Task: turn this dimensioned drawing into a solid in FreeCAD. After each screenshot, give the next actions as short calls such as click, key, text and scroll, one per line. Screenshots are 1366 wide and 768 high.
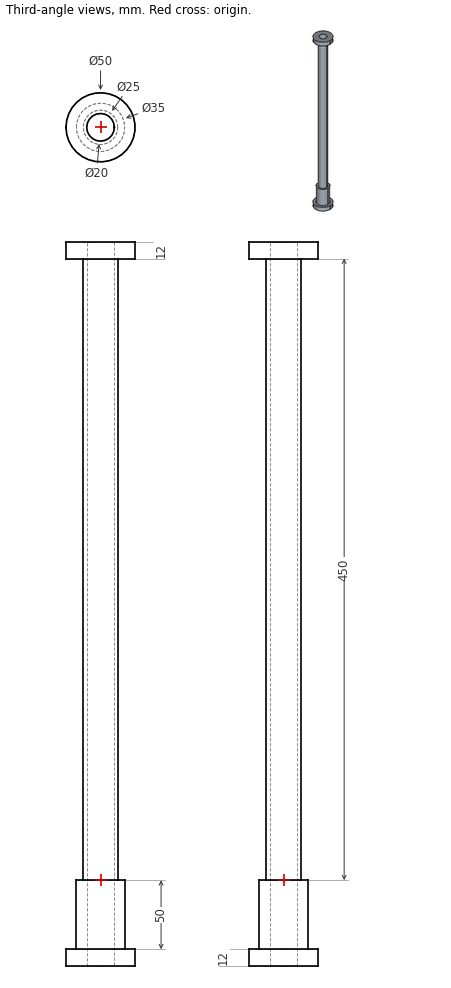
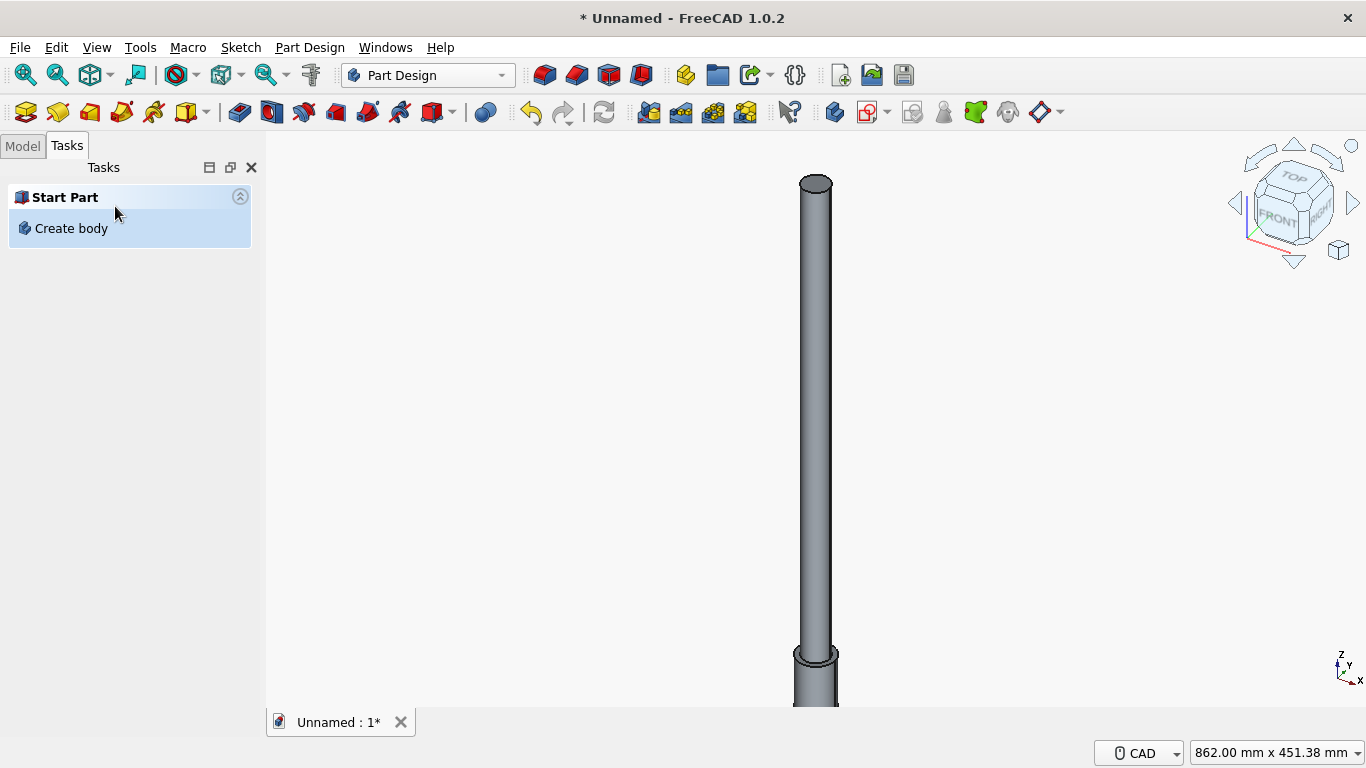
click(26, 76)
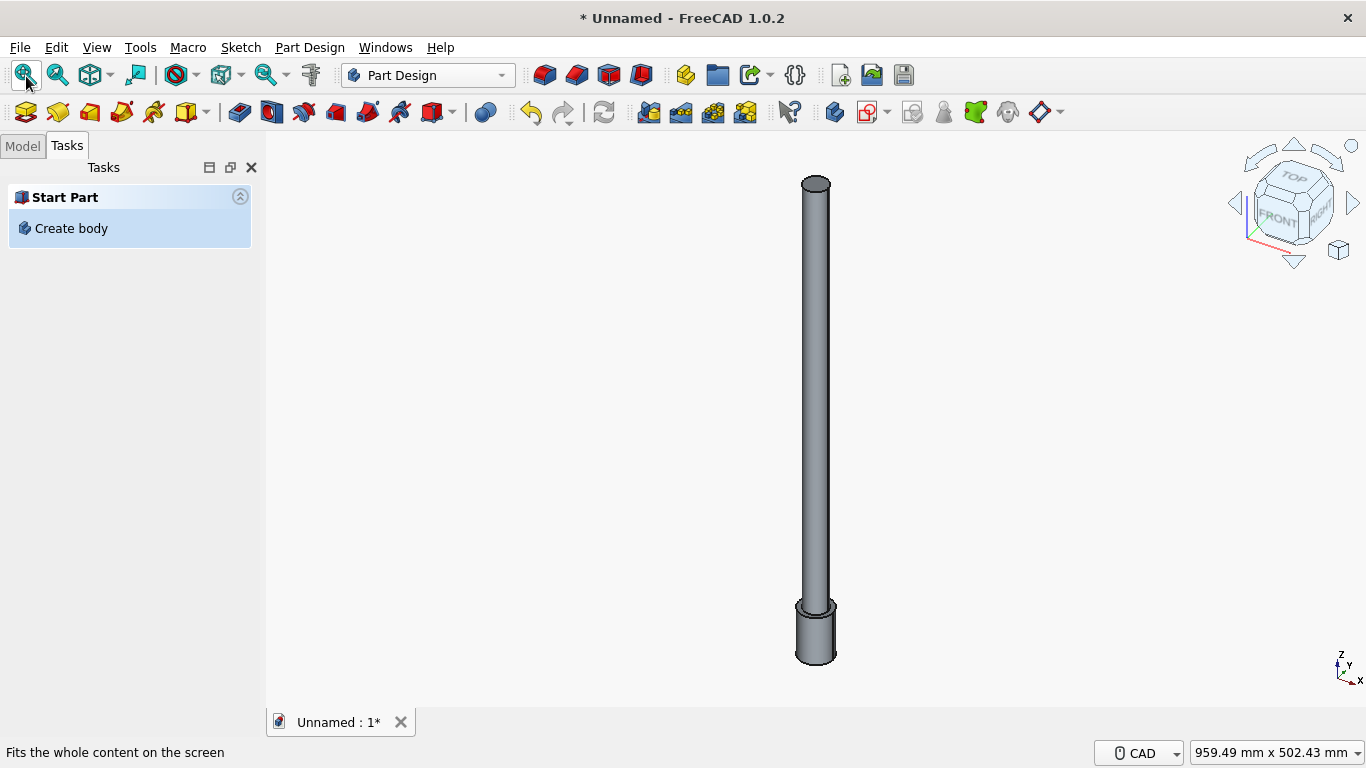
key(5)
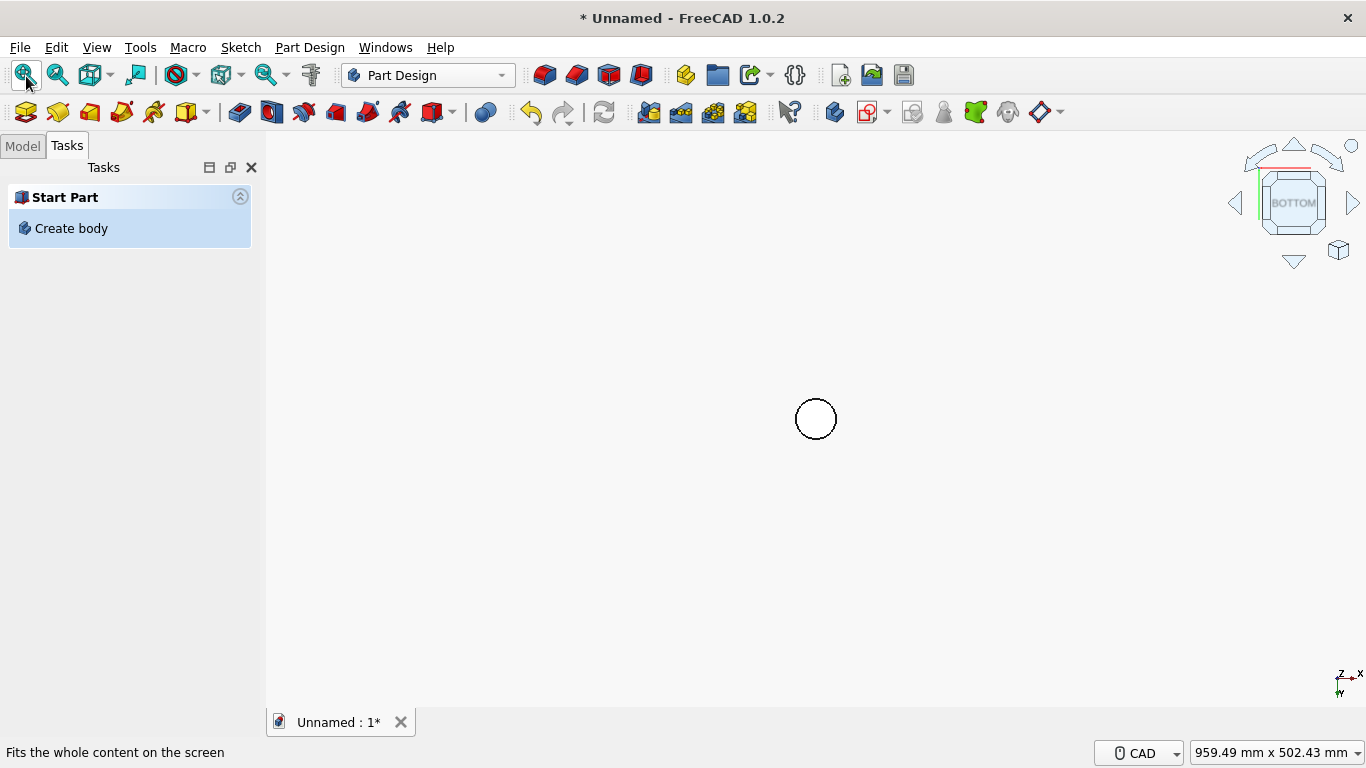
key(v)
key(f)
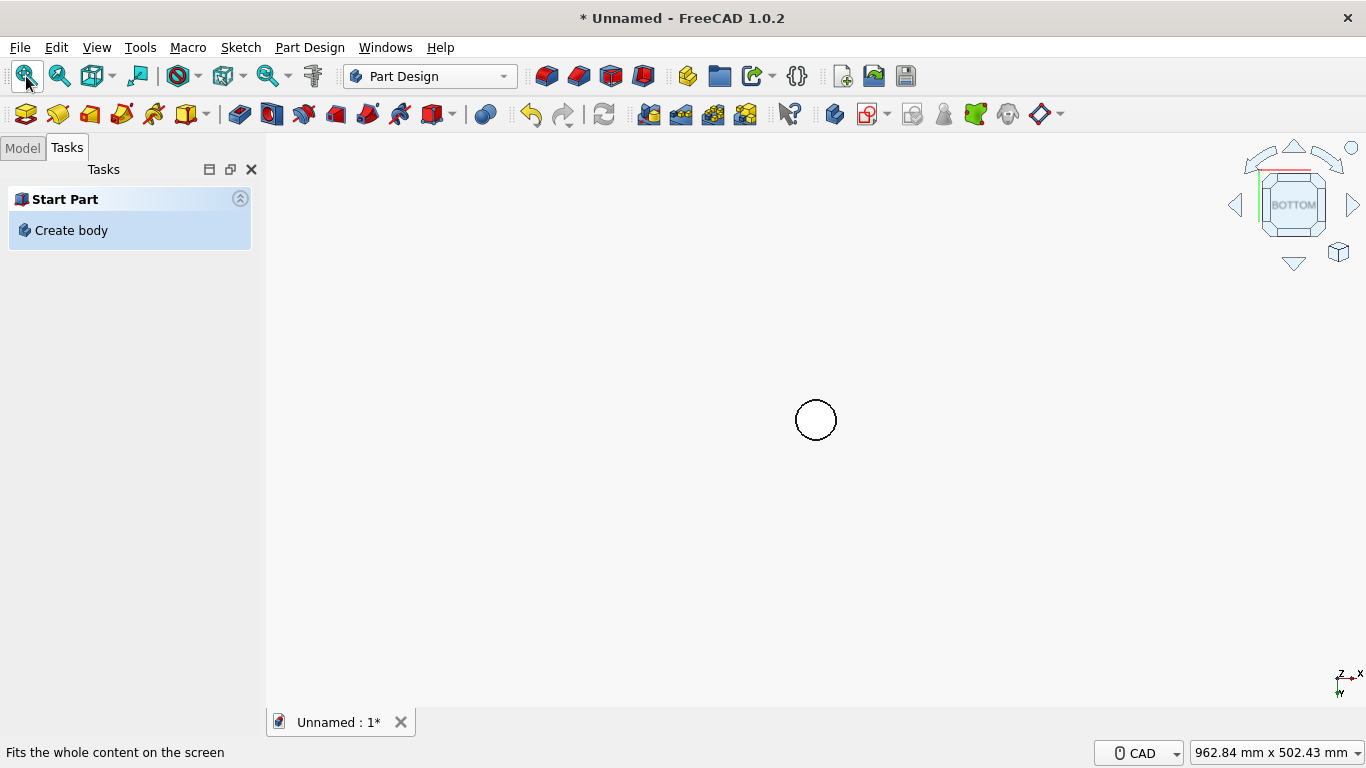
click(816, 419)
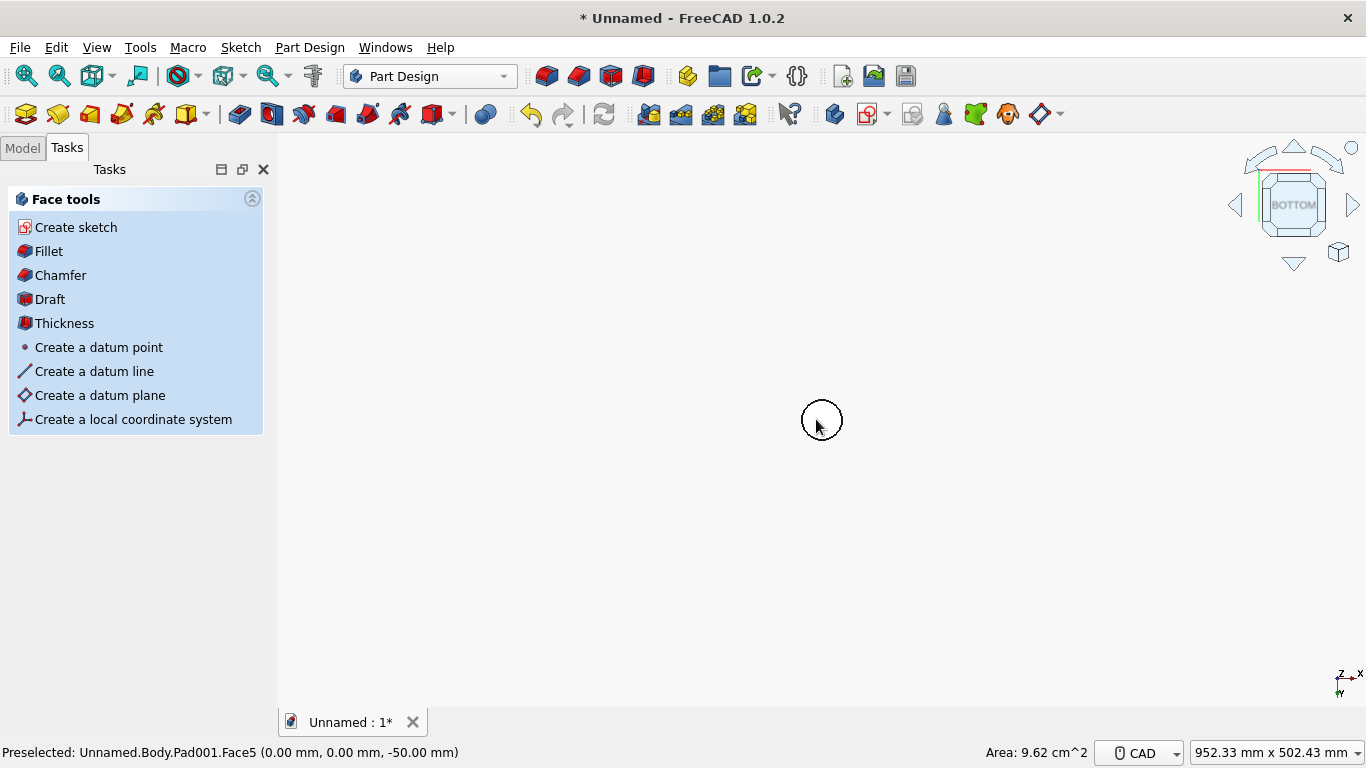
click(868, 114)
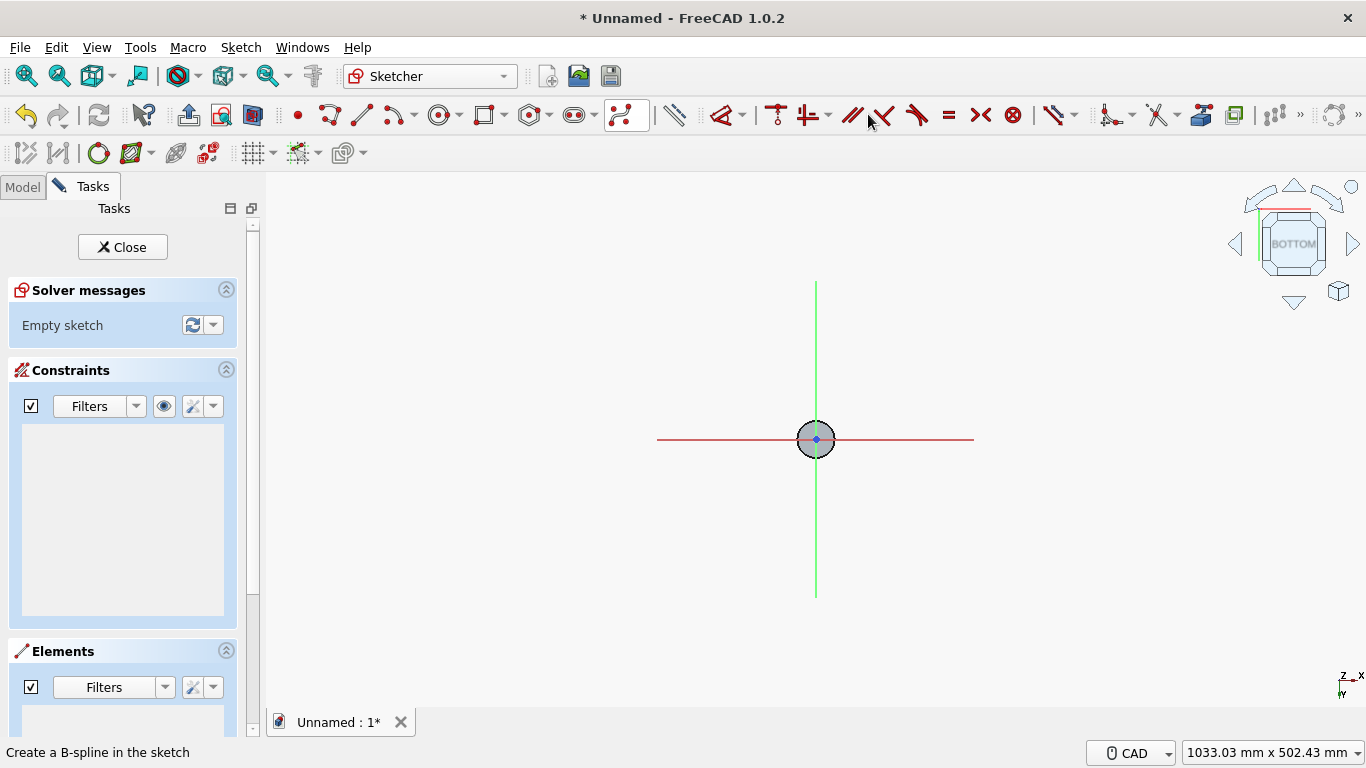
scroll(830, 440, up, 9)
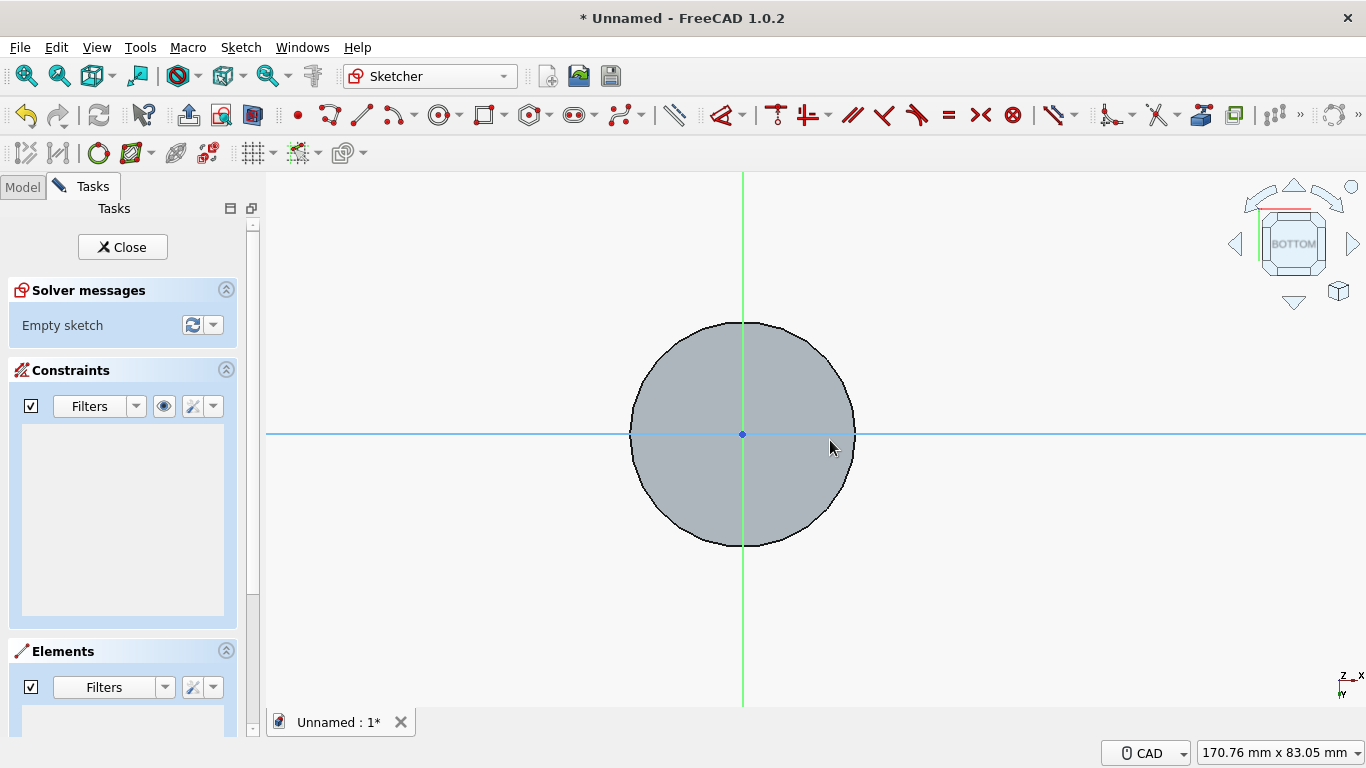
click(440, 116)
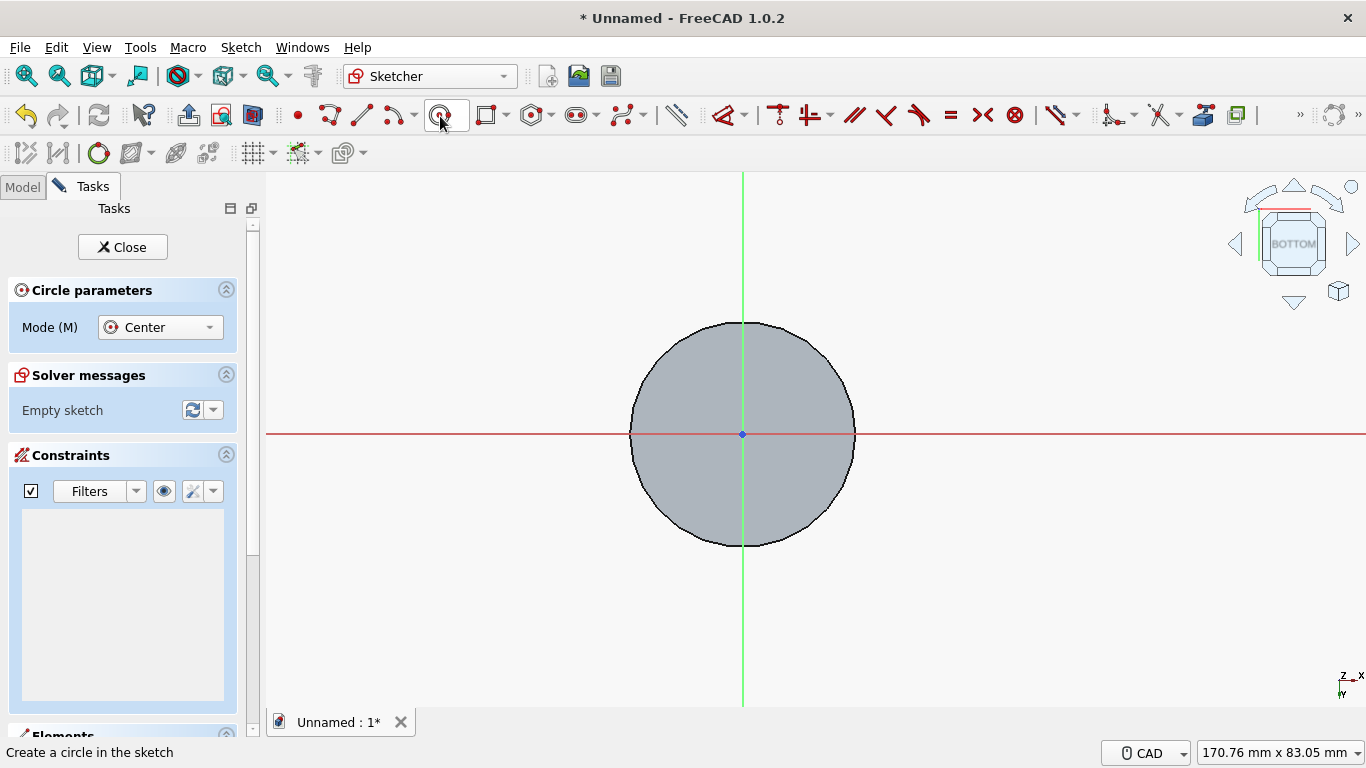
click(743, 434)
click(857, 321)
key(Escape)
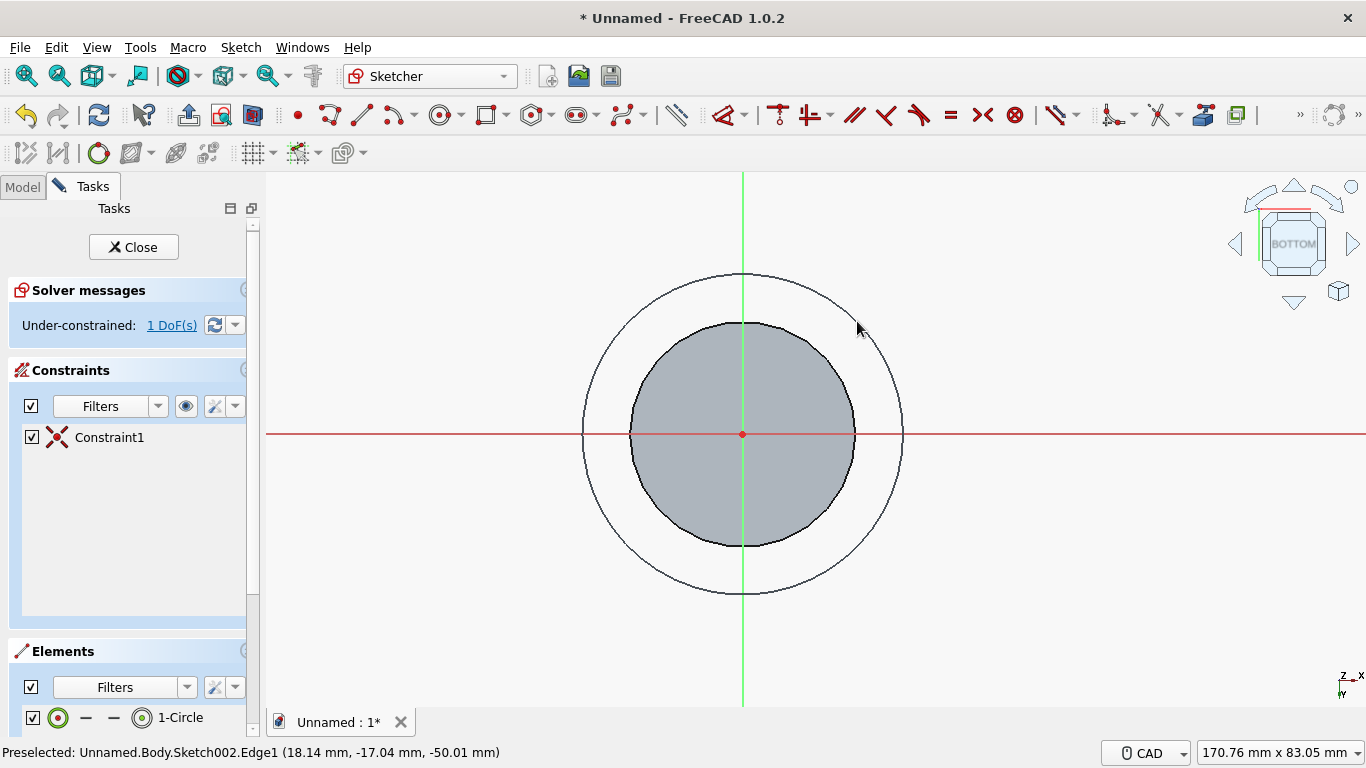
click(724, 116)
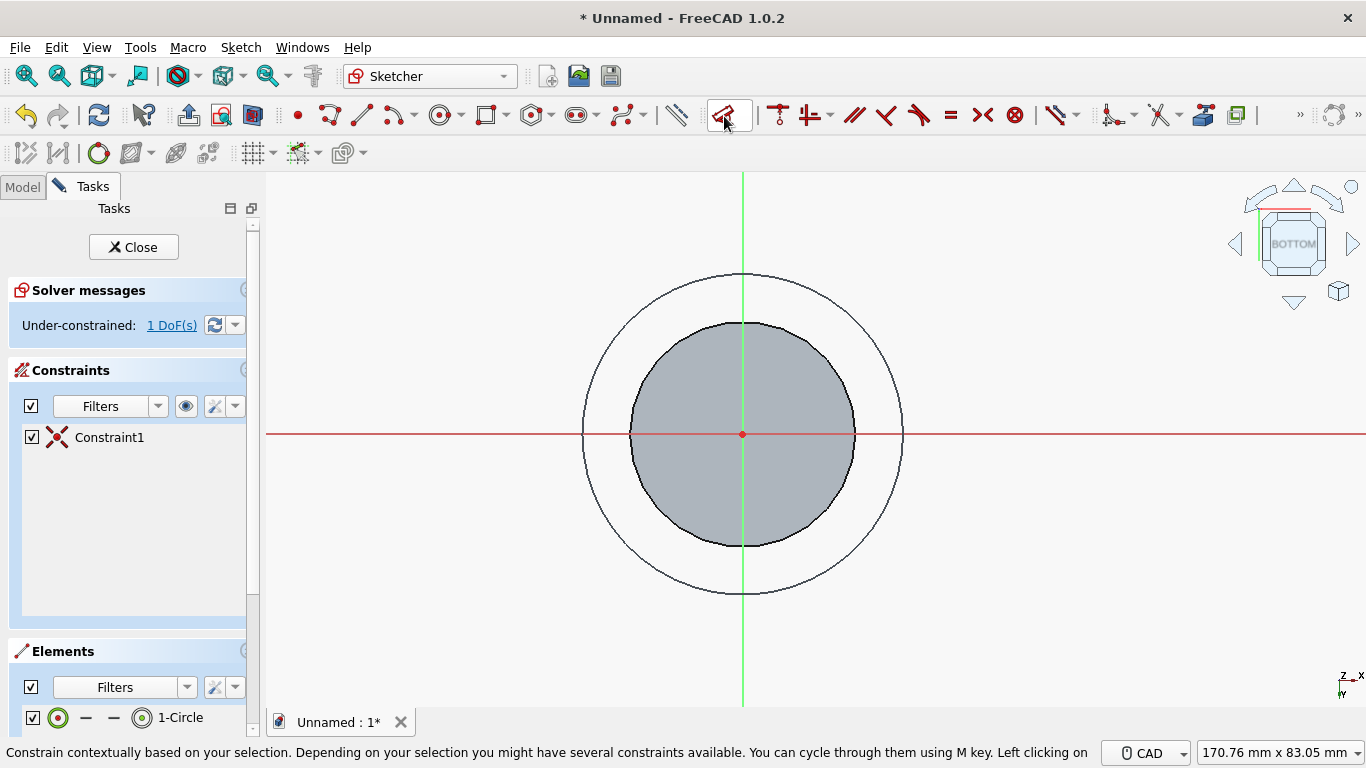
click(856, 321)
click(879, 298)